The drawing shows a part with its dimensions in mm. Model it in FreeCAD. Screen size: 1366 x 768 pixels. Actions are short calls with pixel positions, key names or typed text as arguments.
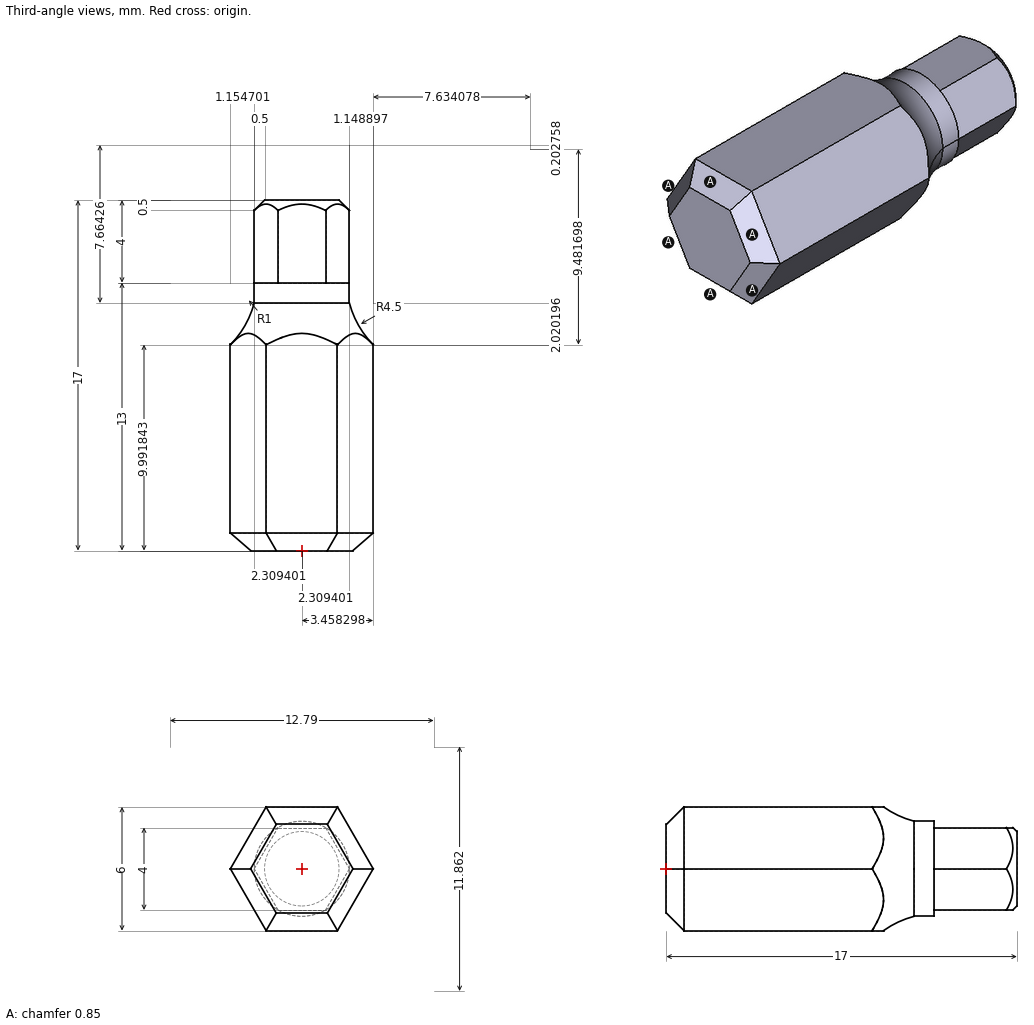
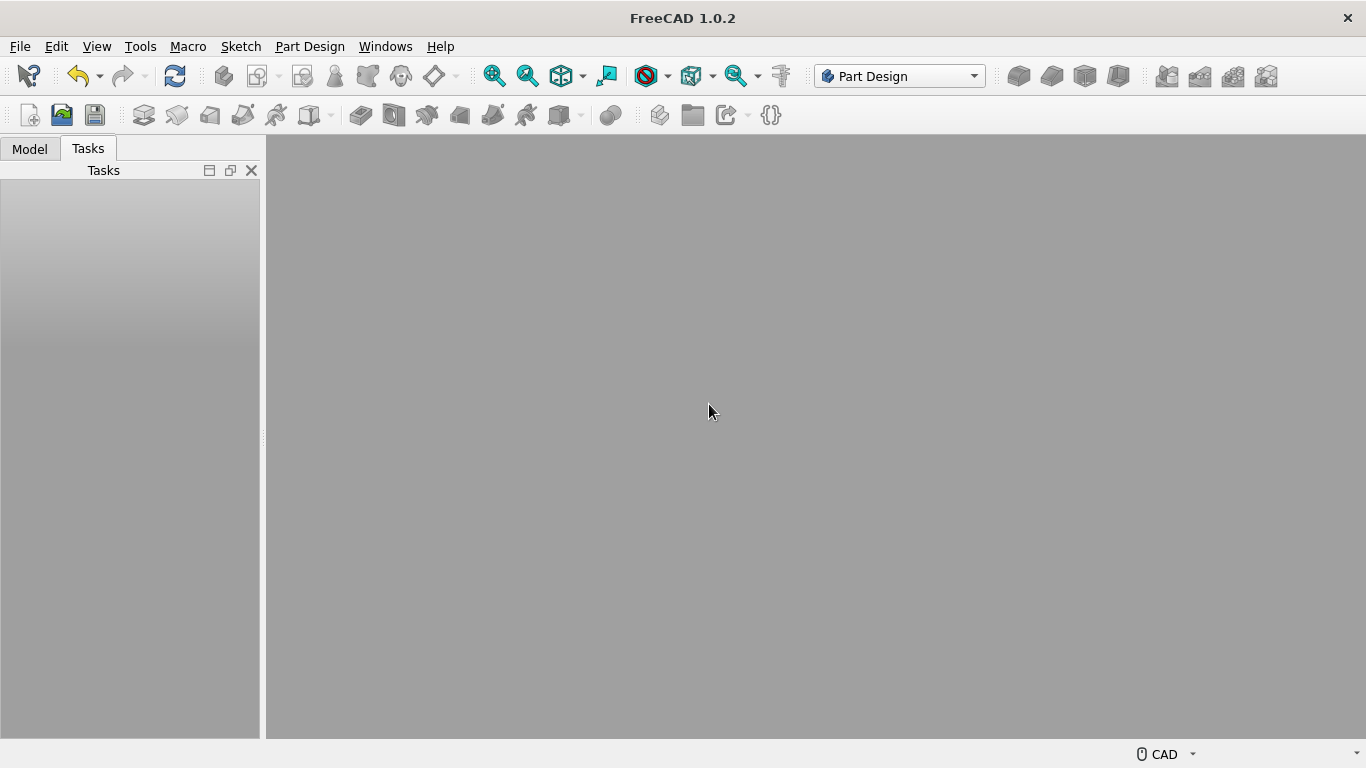
click(29, 116)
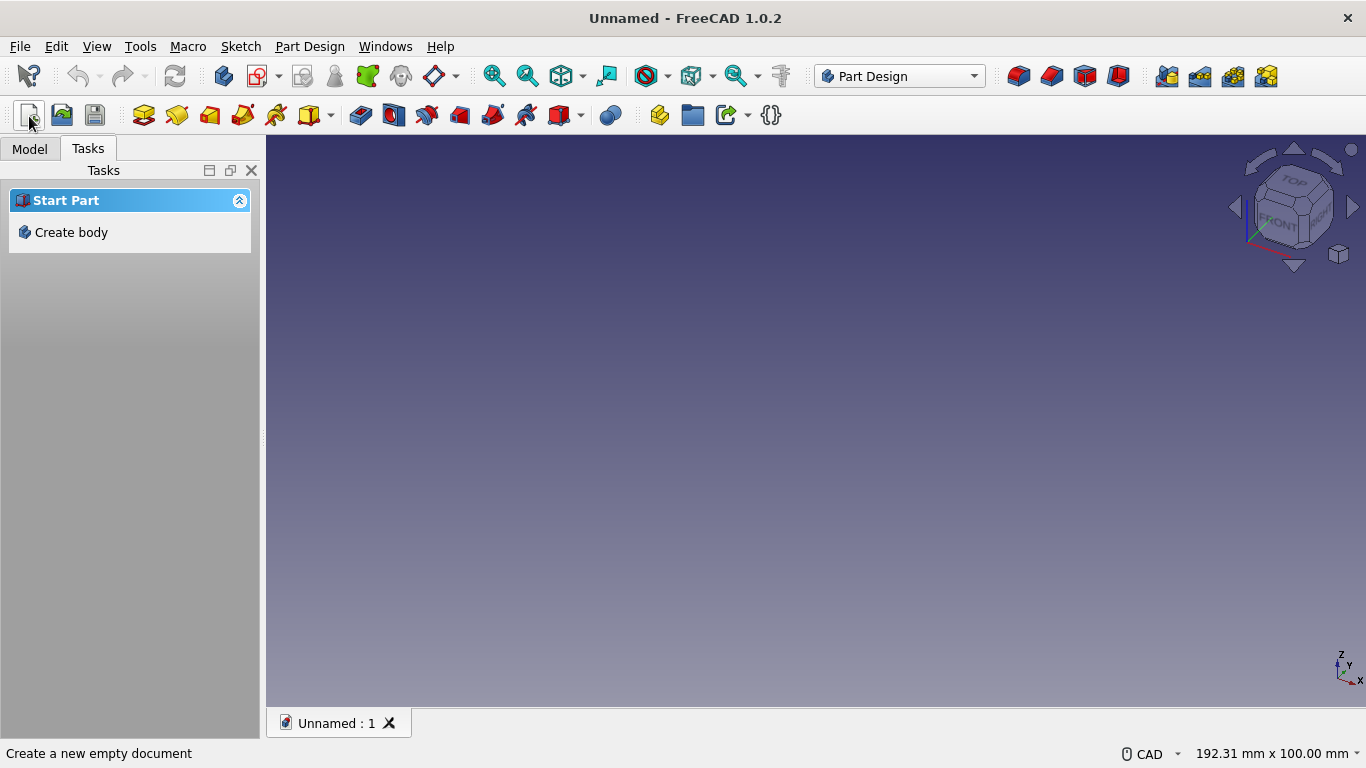
click(256, 76)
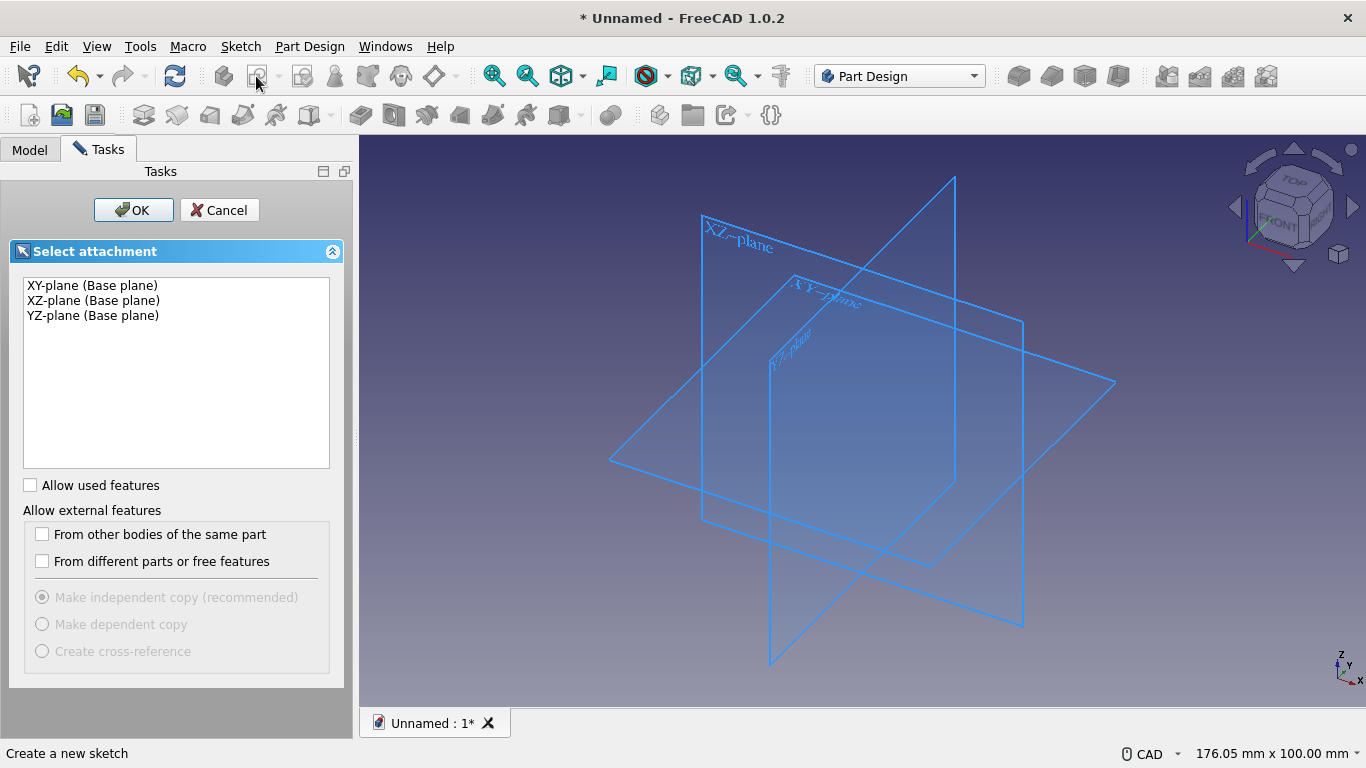
click(84, 300)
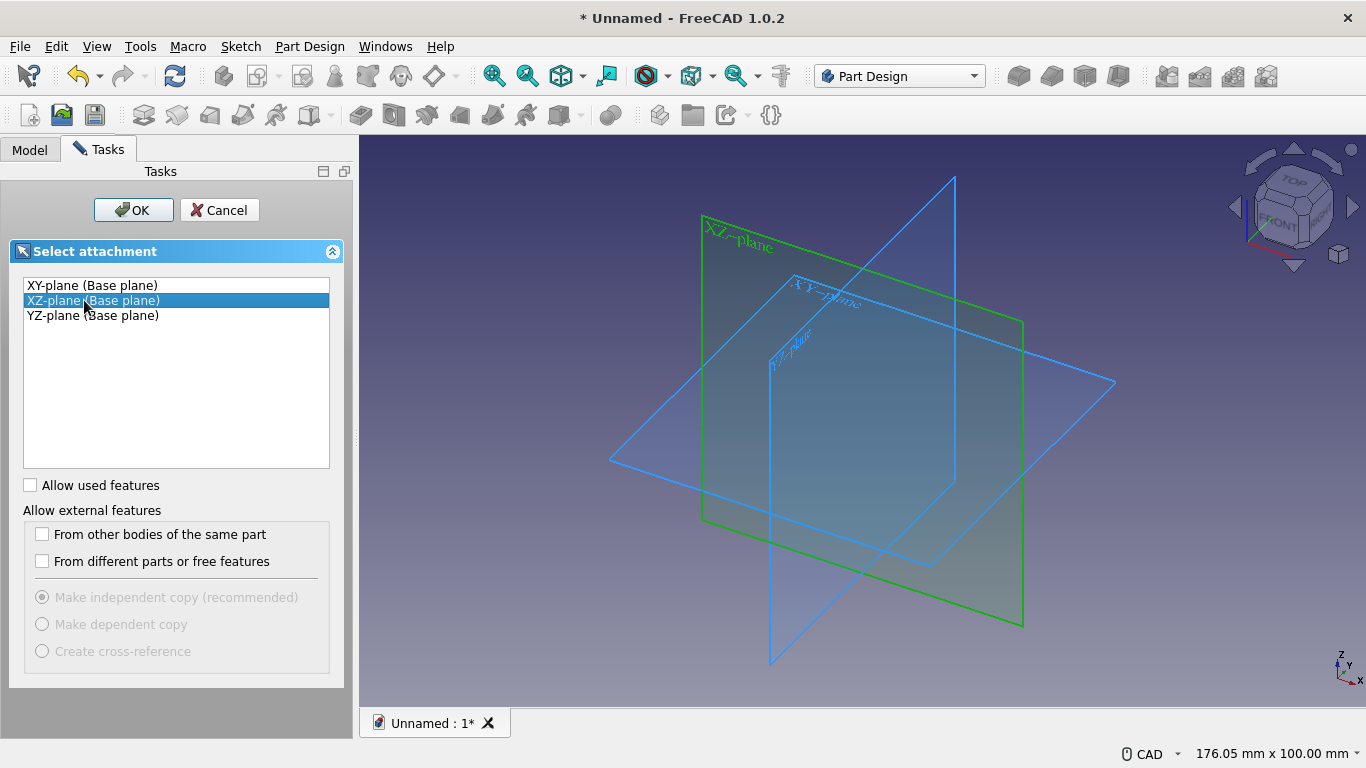
click(134, 210)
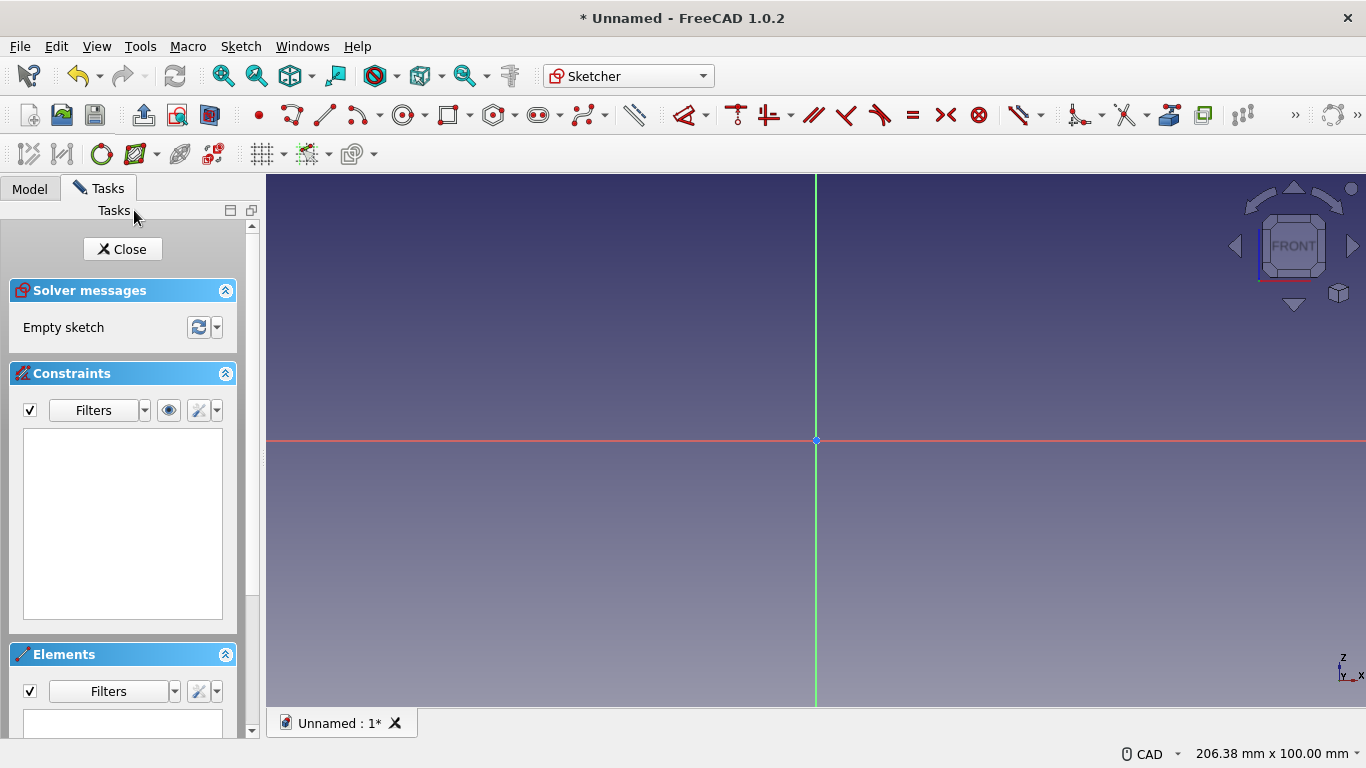
scroll(823, 440, up, 12)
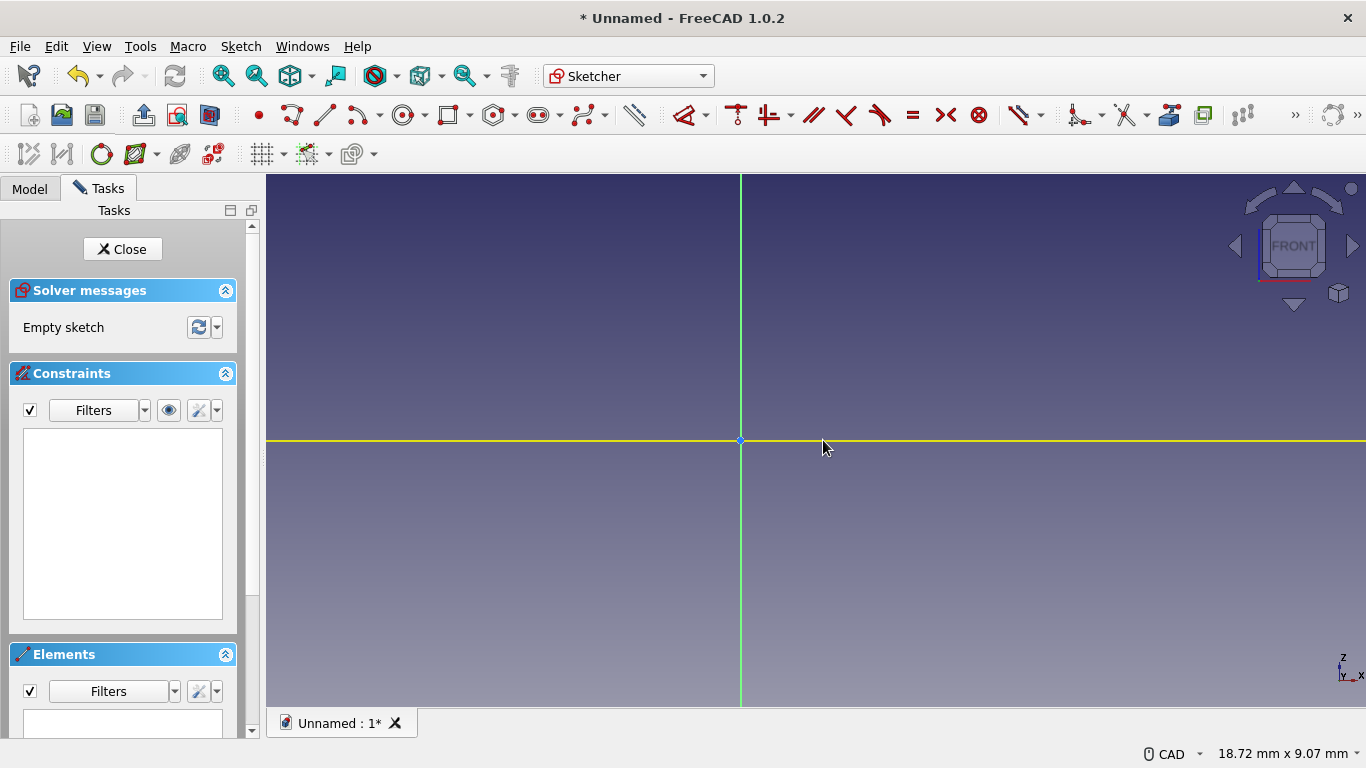
click(492, 116)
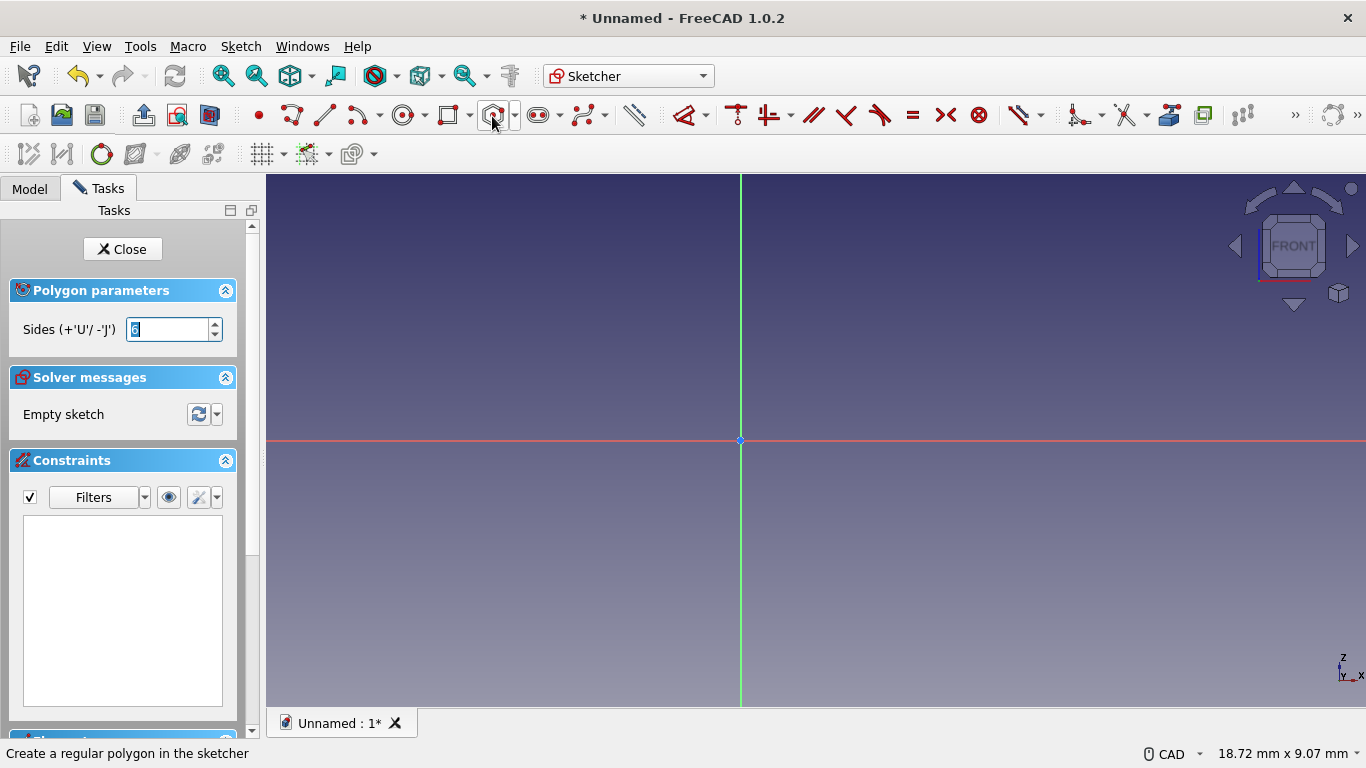
click(741, 440)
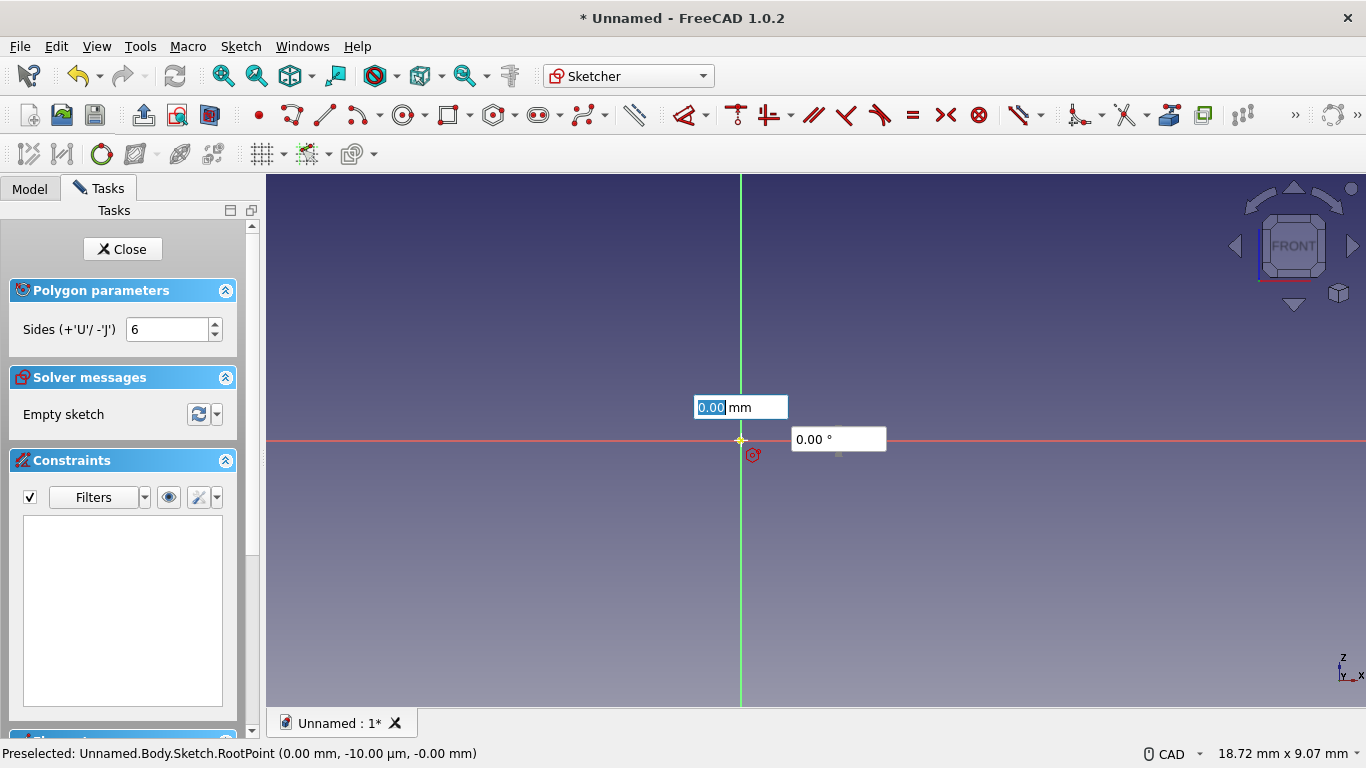
click(944, 440)
key(Escape)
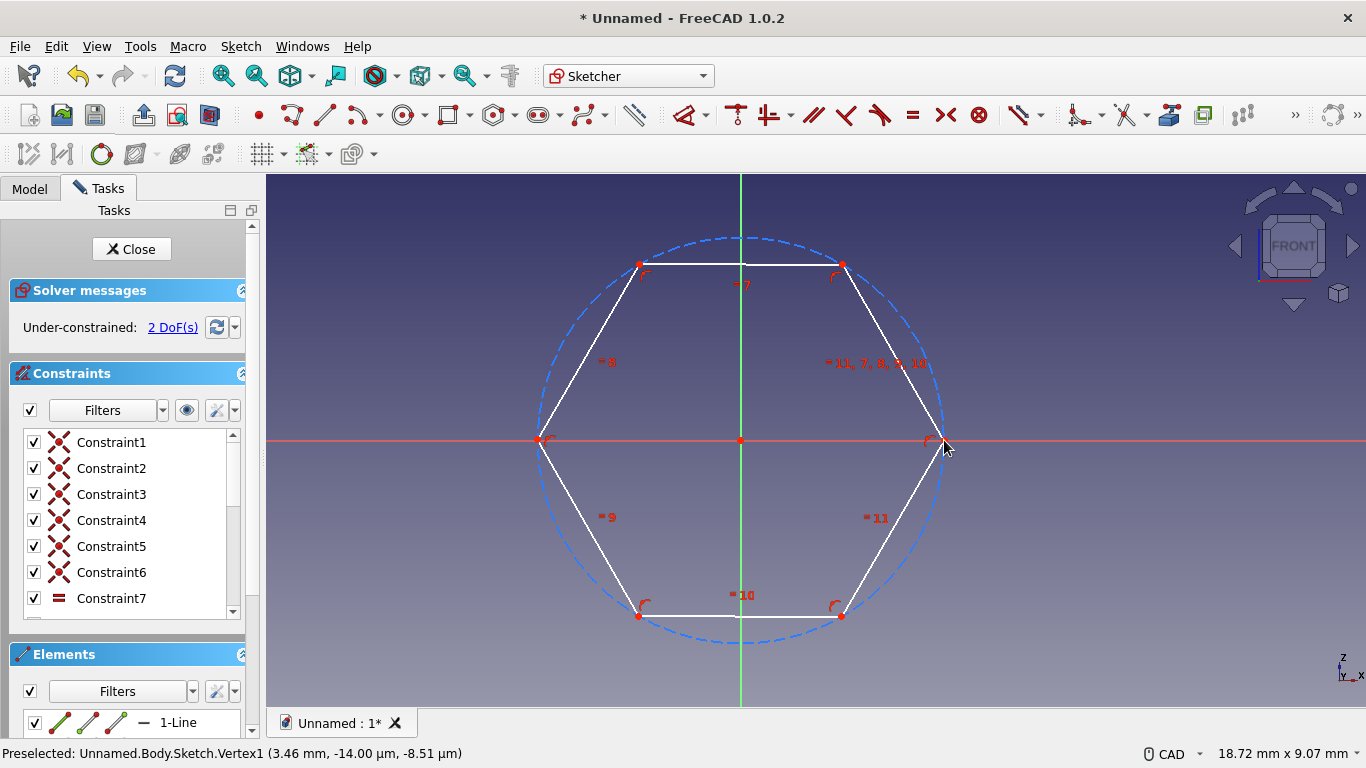
click(782, 265)